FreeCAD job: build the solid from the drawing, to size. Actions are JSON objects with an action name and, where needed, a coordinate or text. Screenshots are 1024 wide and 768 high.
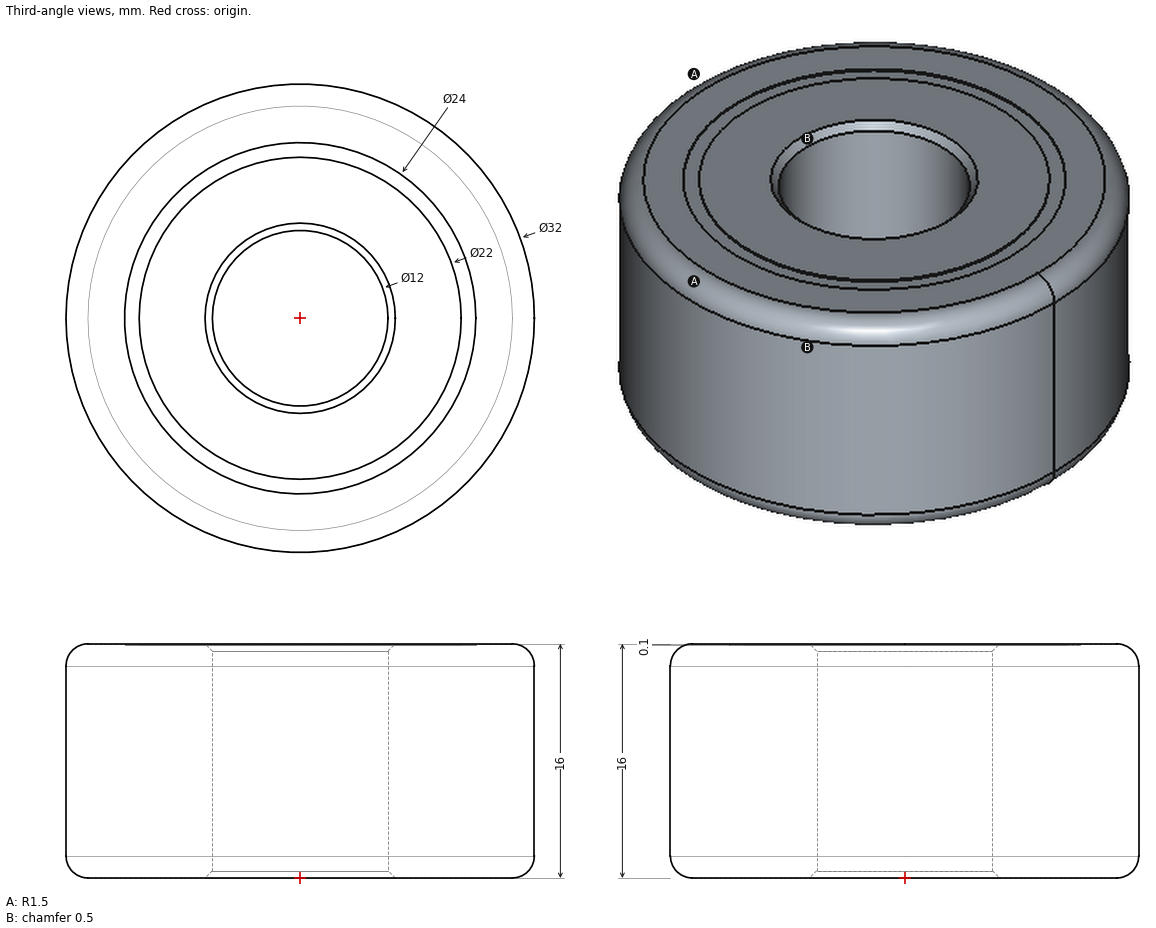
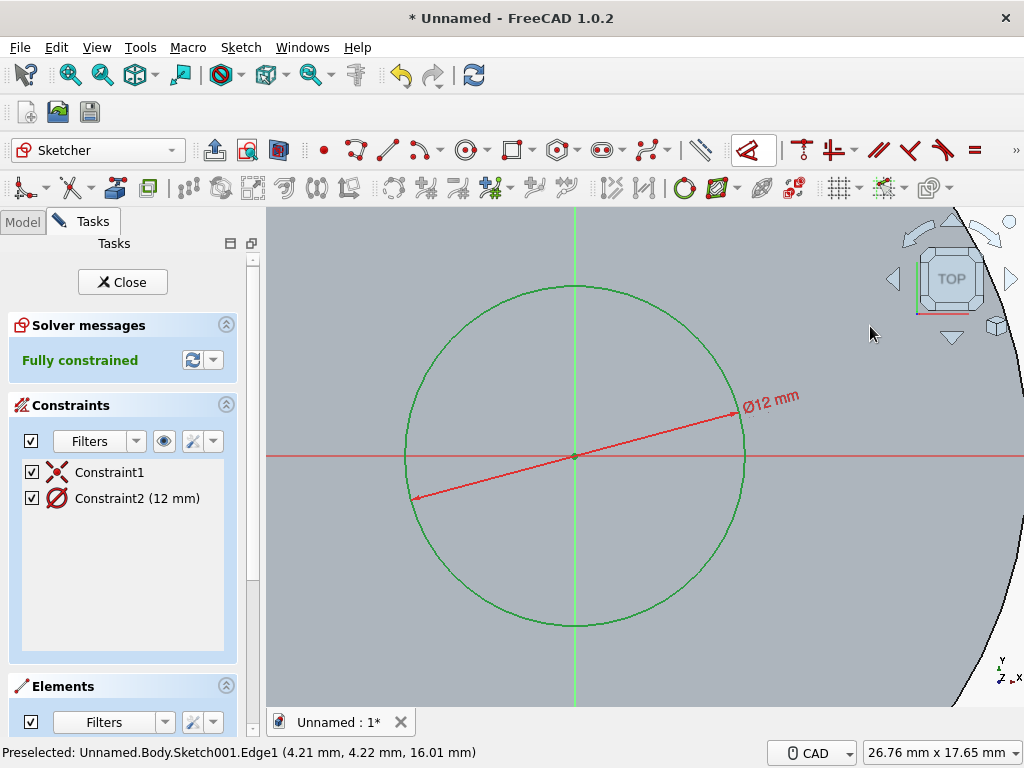
{"action": "left_click", "coordinate": [123, 282]}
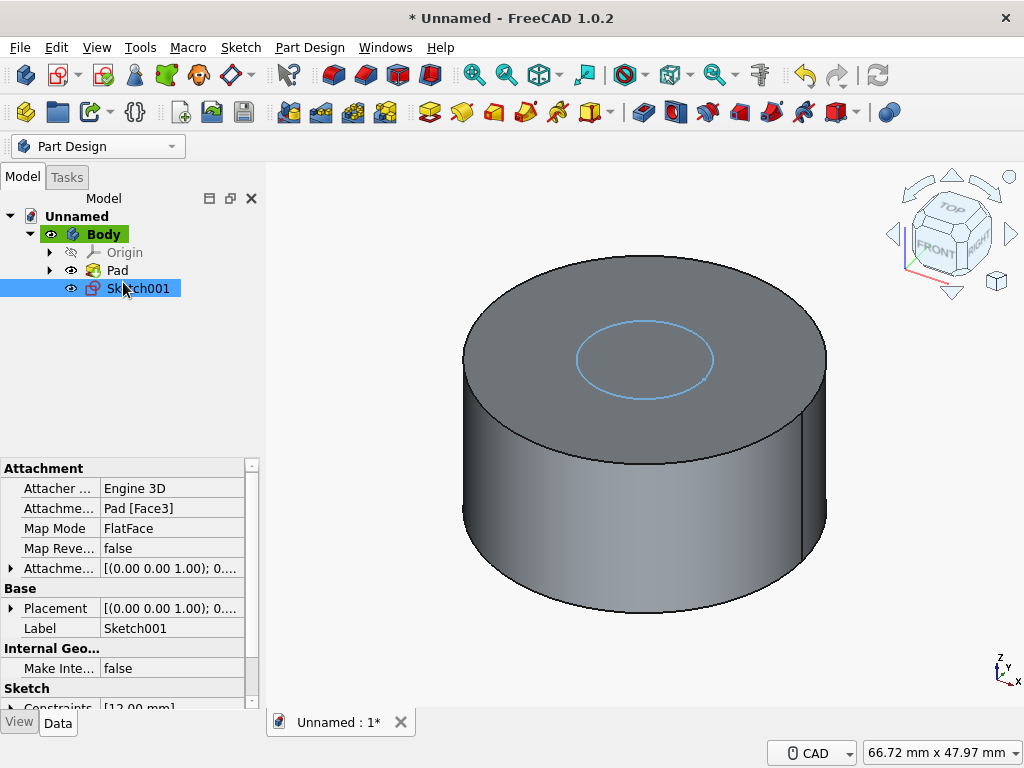
{"action": "left_click", "coordinate": [644, 112]}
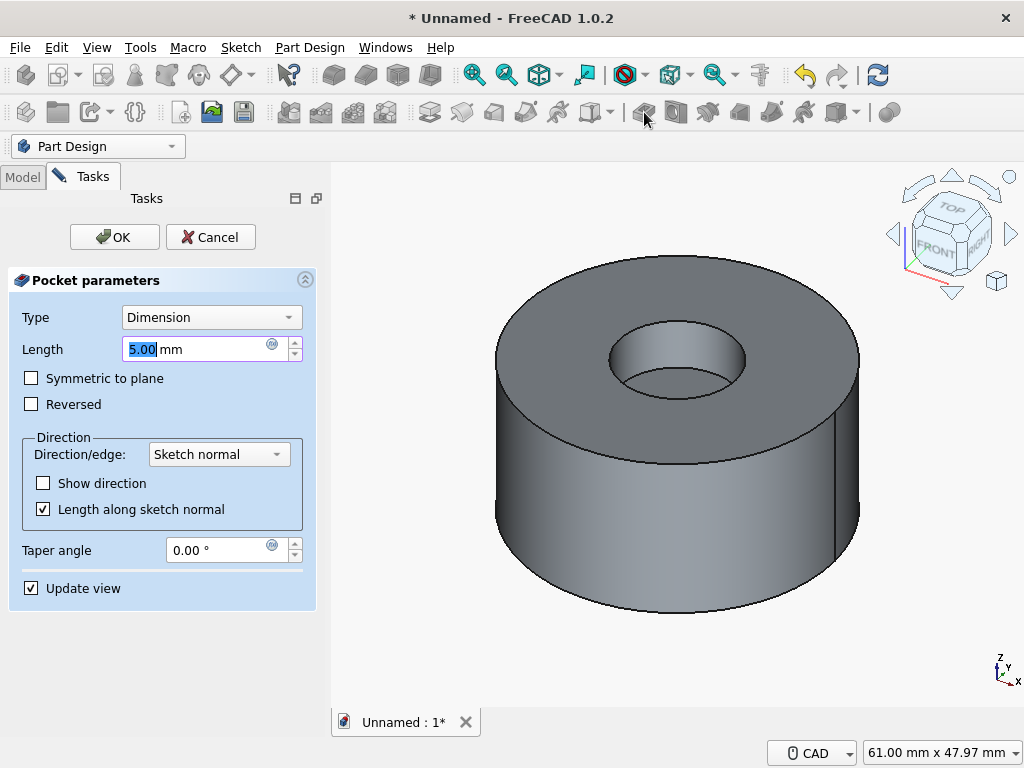
{"action": "type", "text": "16"}
{"action": "key", "text": "Tab"}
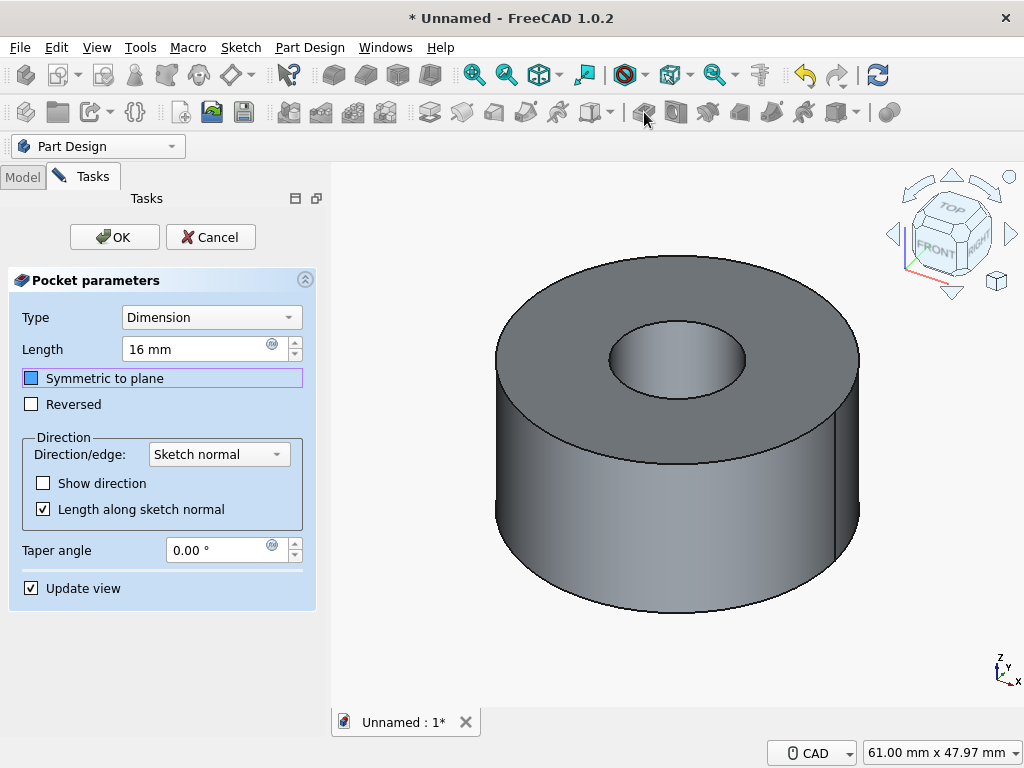
{"action": "left_click", "coordinate": [115, 237]}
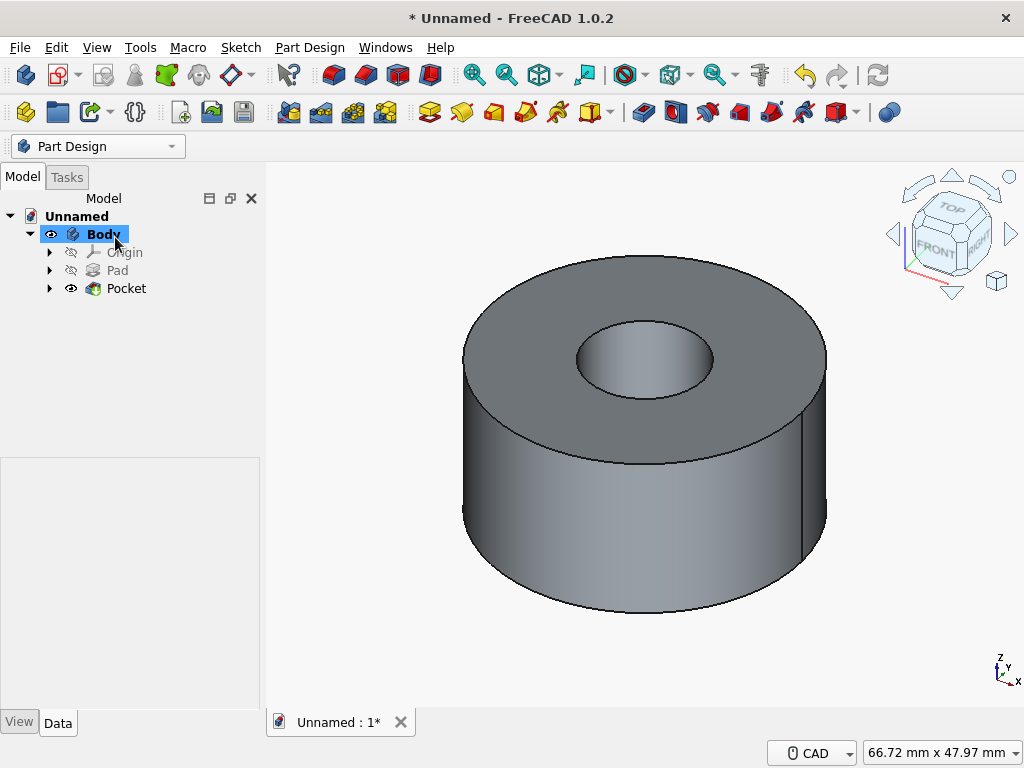
{"action": "left_click", "coordinate": [742, 322]}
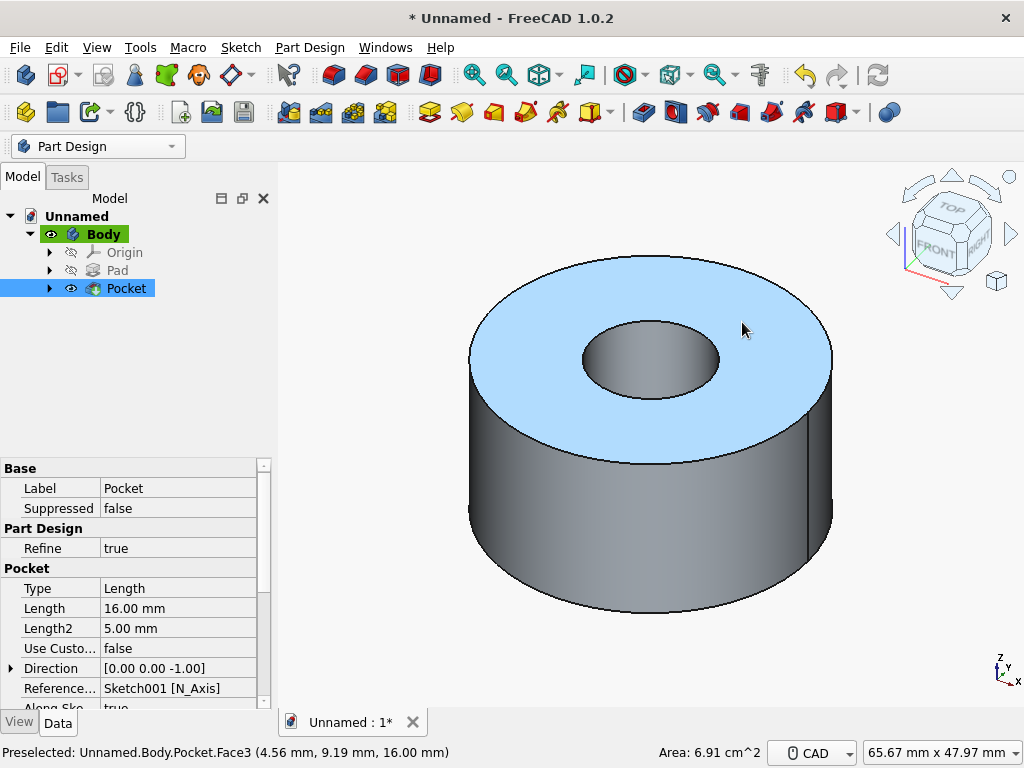
{"action": "left_click", "coordinate": [58, 76]}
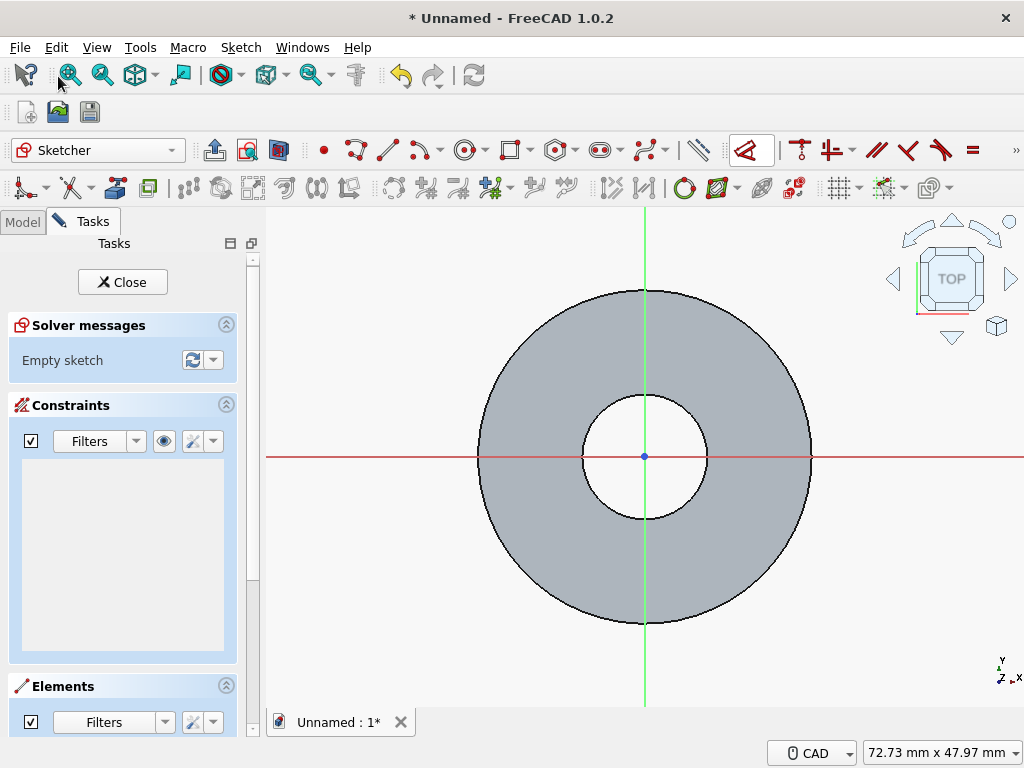
{"action": "left_click", "coordinate": [466, 150]}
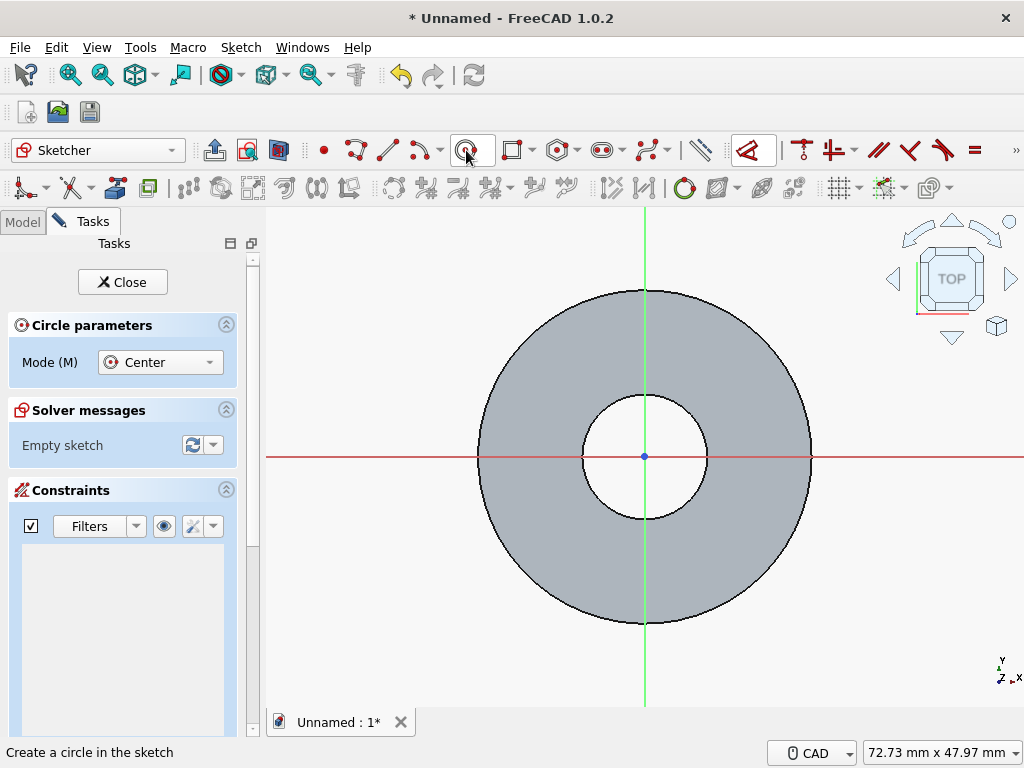
{"action": "left_click", "coordinate": [645, 457]}
{"action": "left_click", "coordinate": [733, 369]}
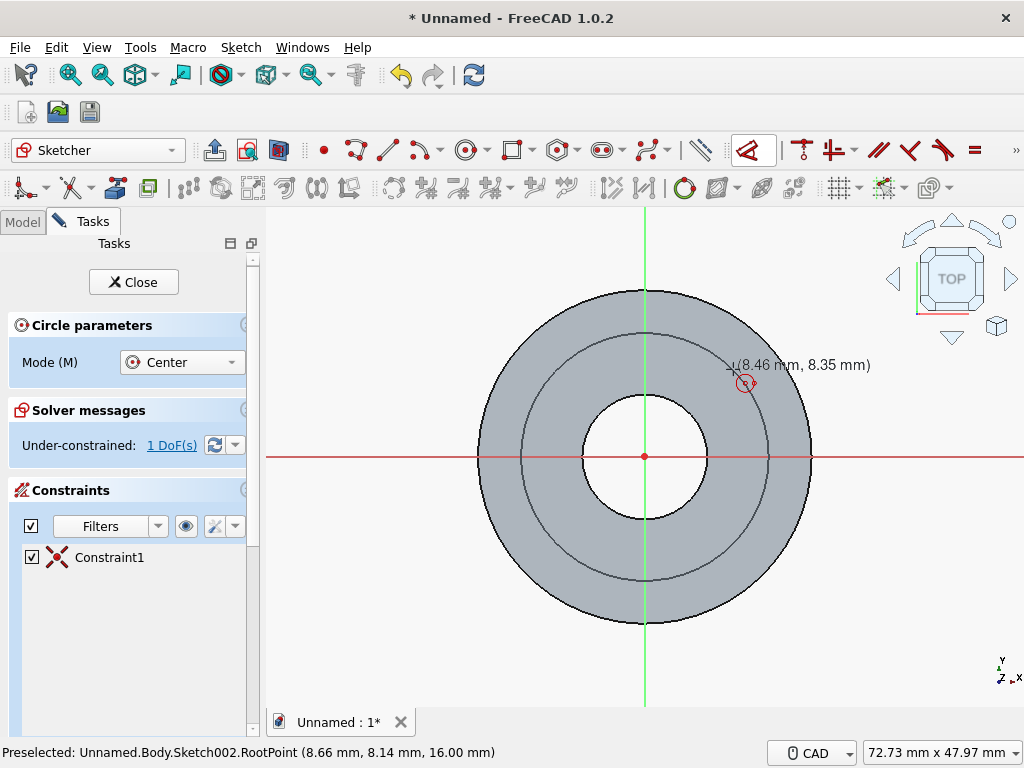
{"action": "left_click", "coordinate": [645, 457]}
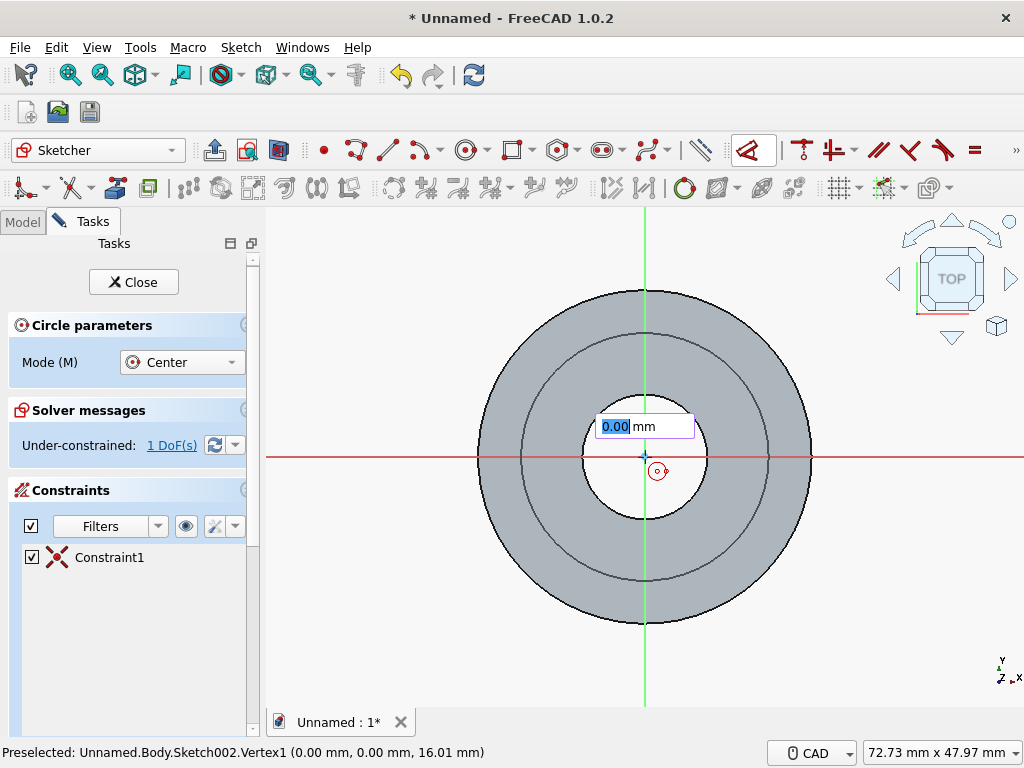
{"action": "scroll", "coordinate": [726, 376], "scroll_direction": "up", "scroll_amount": 3}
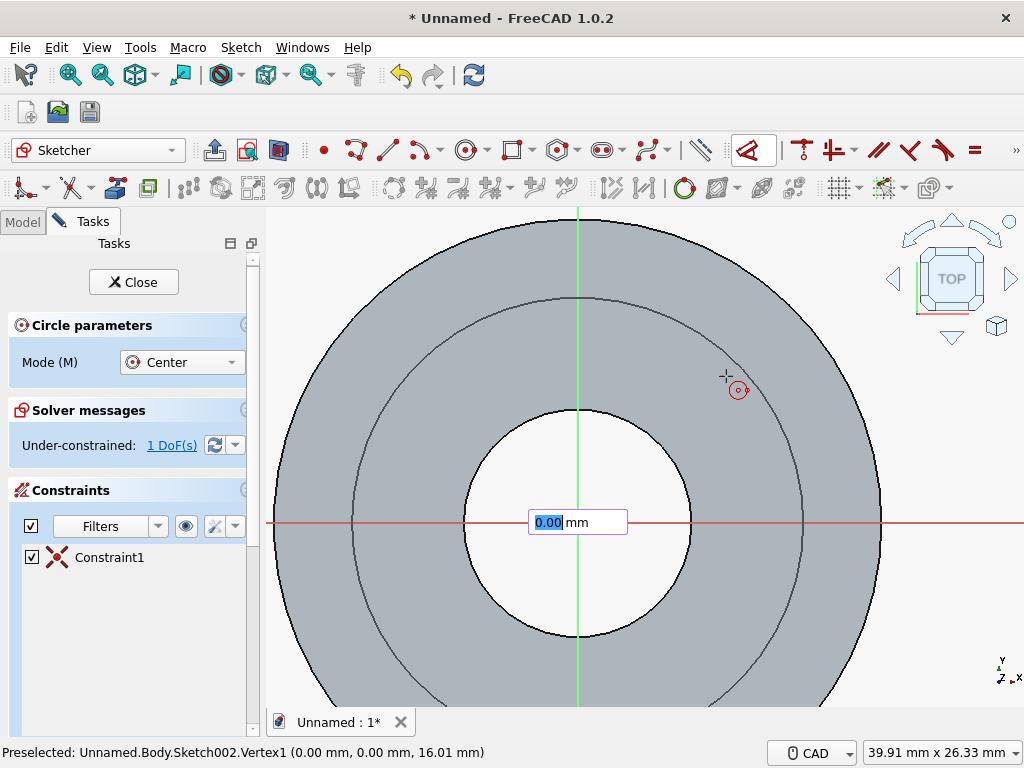
{"action": "left_click", "coordinate": [725, 376]}
{"action": "key", "text": "Escape"}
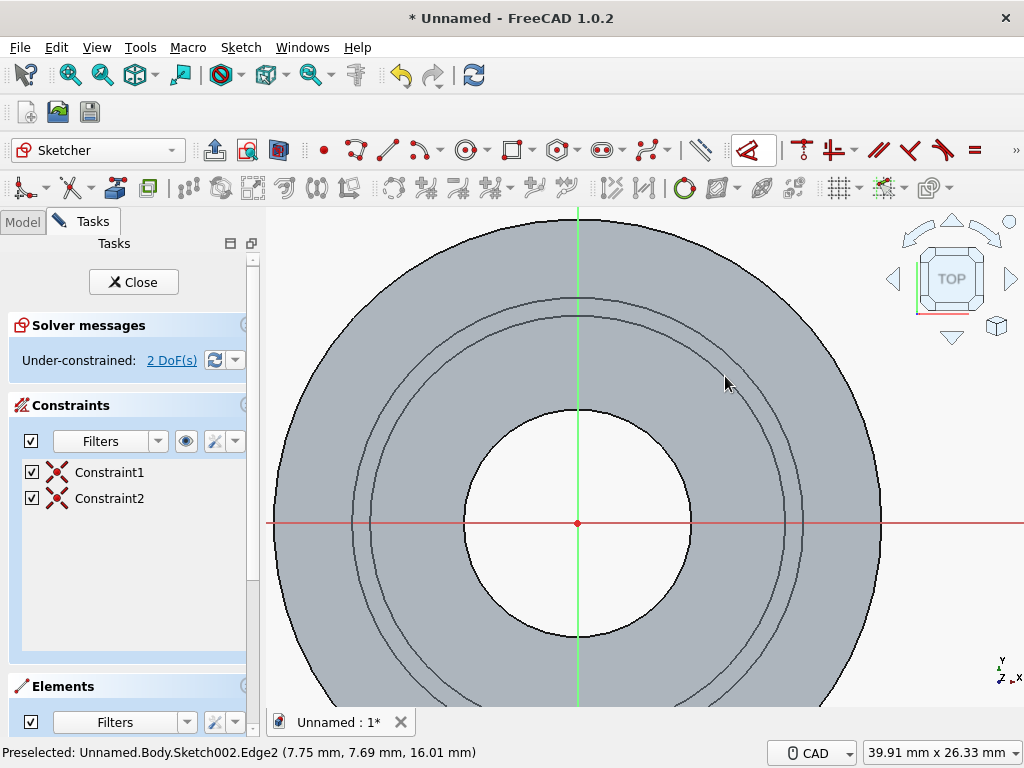
{"action": "left_click", "coordinate": [737, 363]}